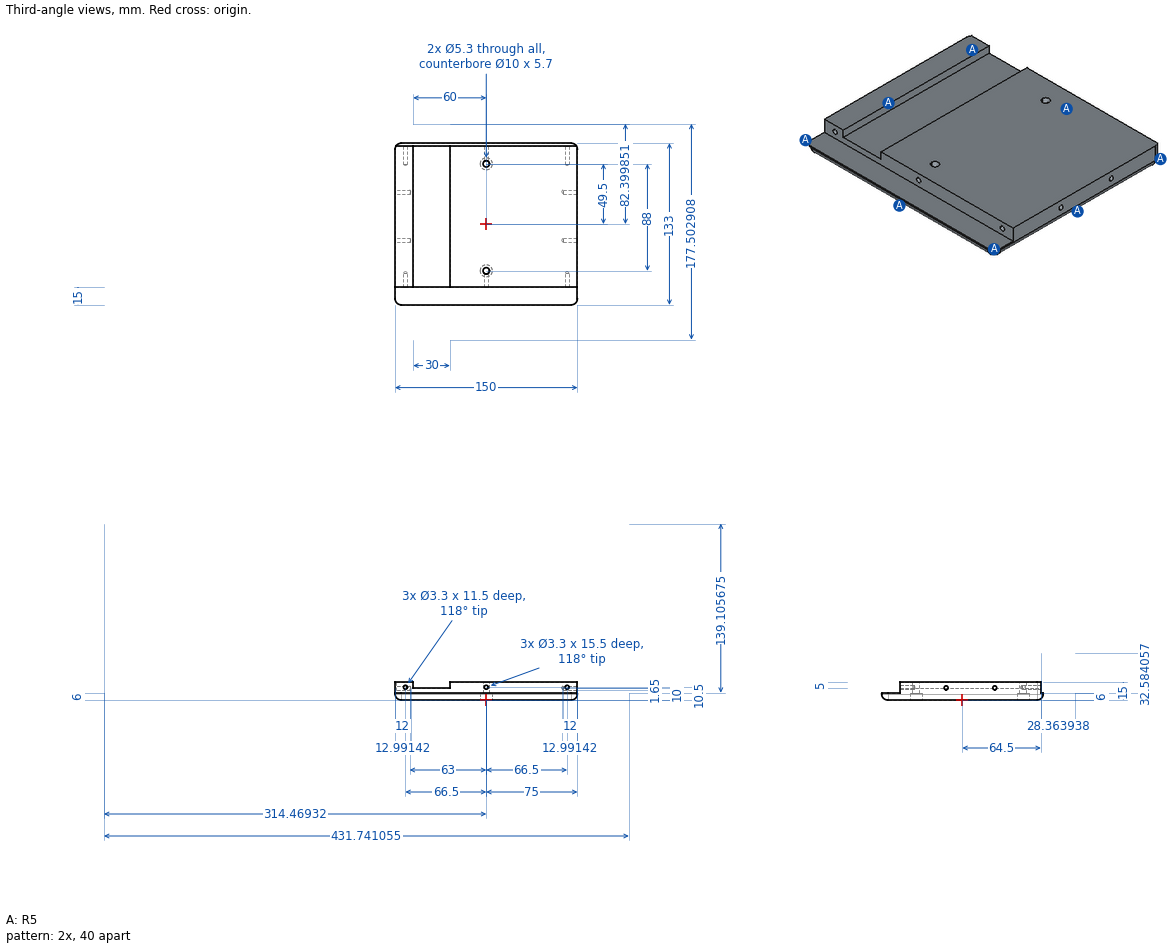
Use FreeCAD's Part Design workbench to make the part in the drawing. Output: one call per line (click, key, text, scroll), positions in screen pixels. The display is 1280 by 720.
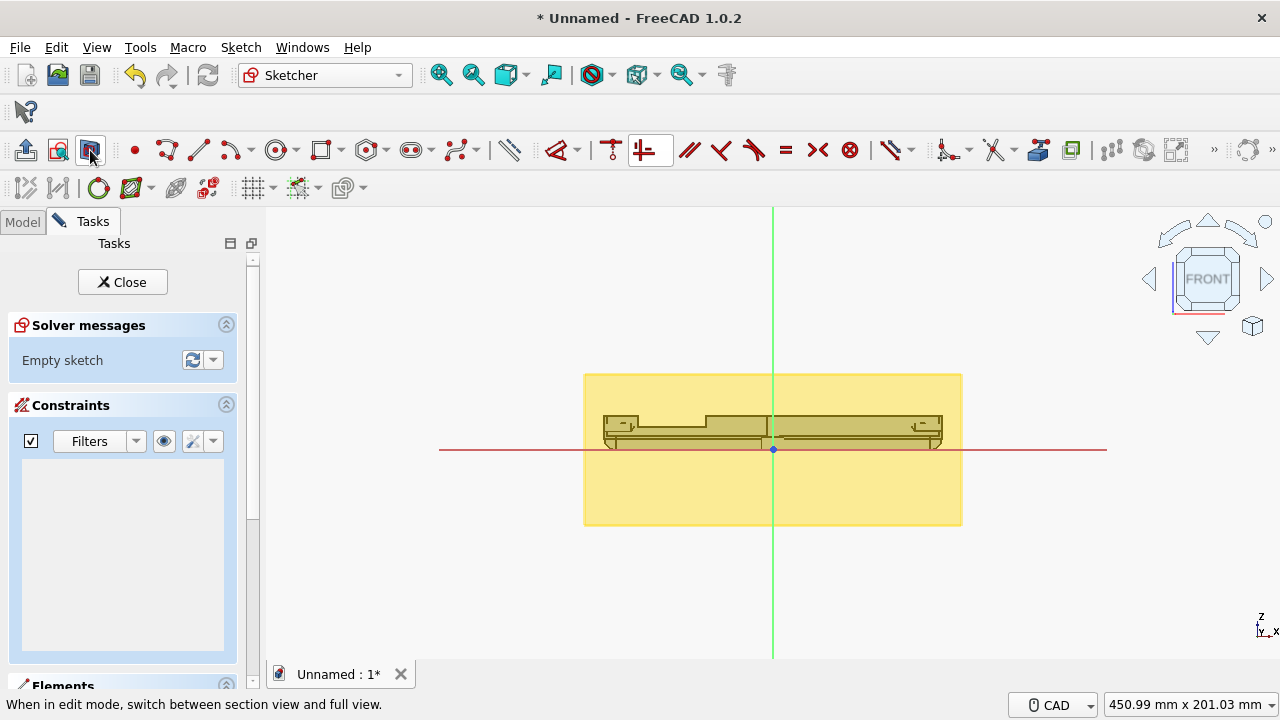
scroll(606, 429, up, 13)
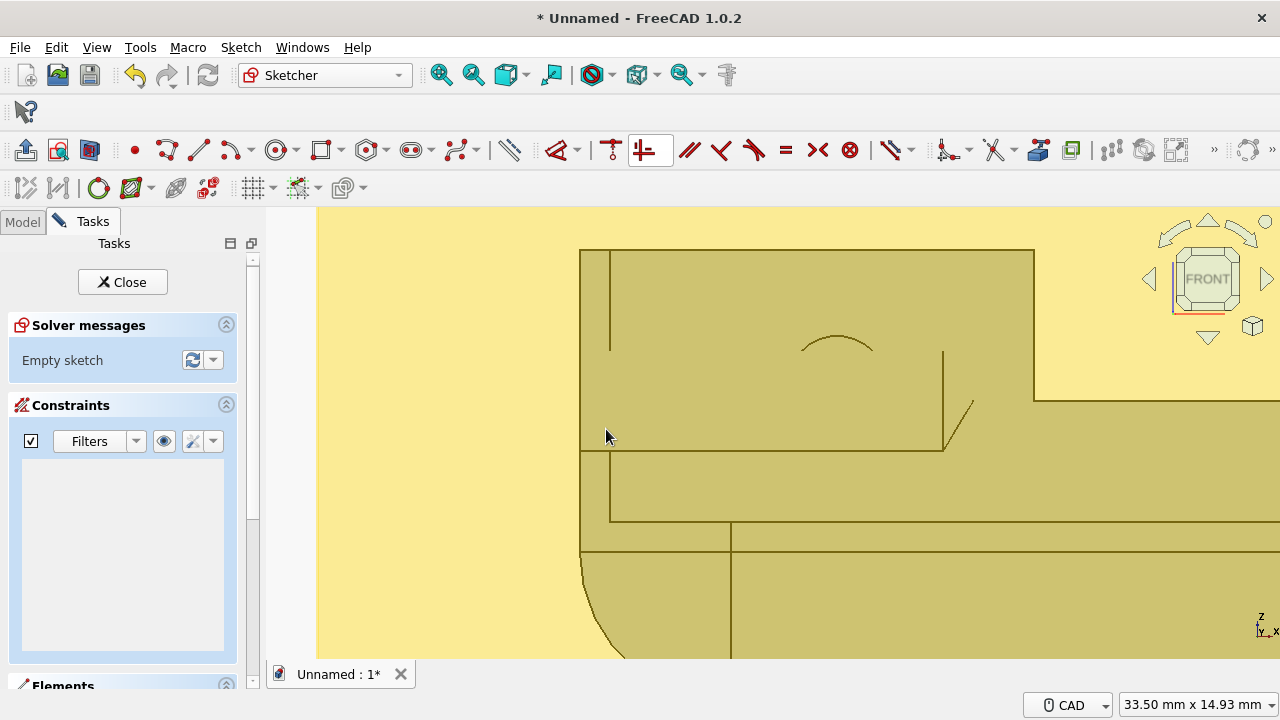
click(168, 150)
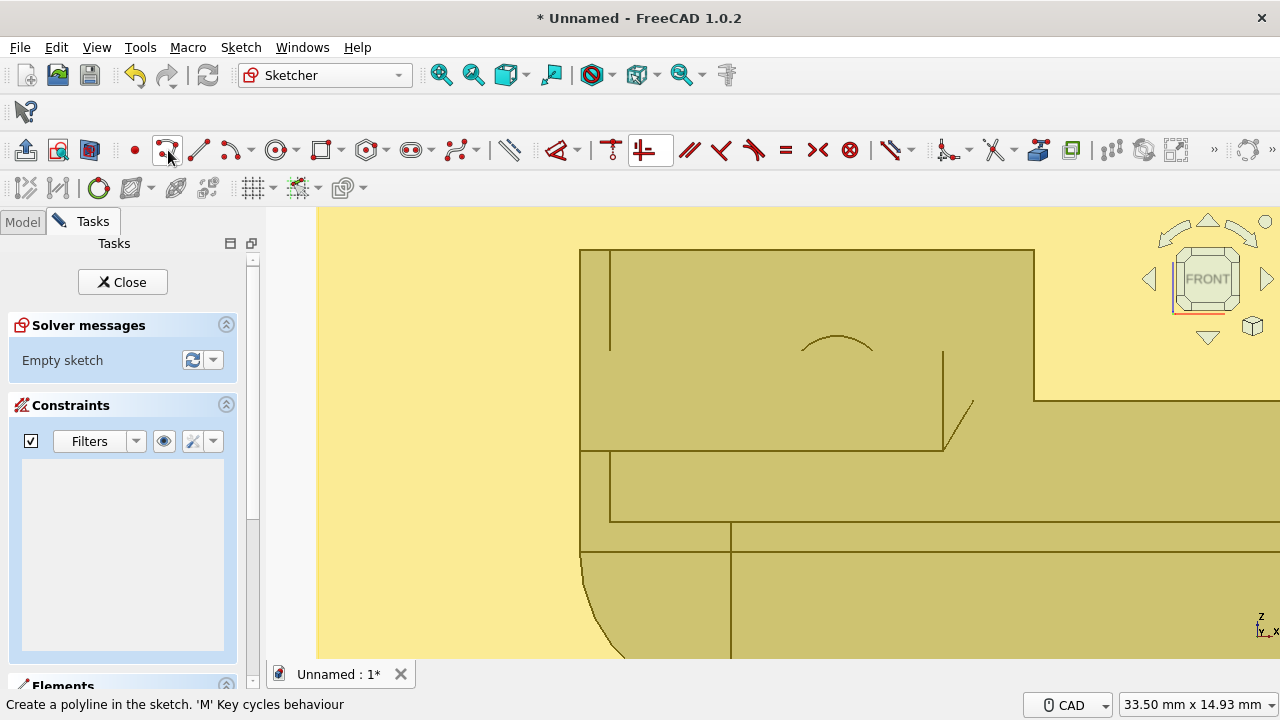
click(973, 401)
click(943, 451)
click(580, 451)
click(580, 401)
click(973, 402)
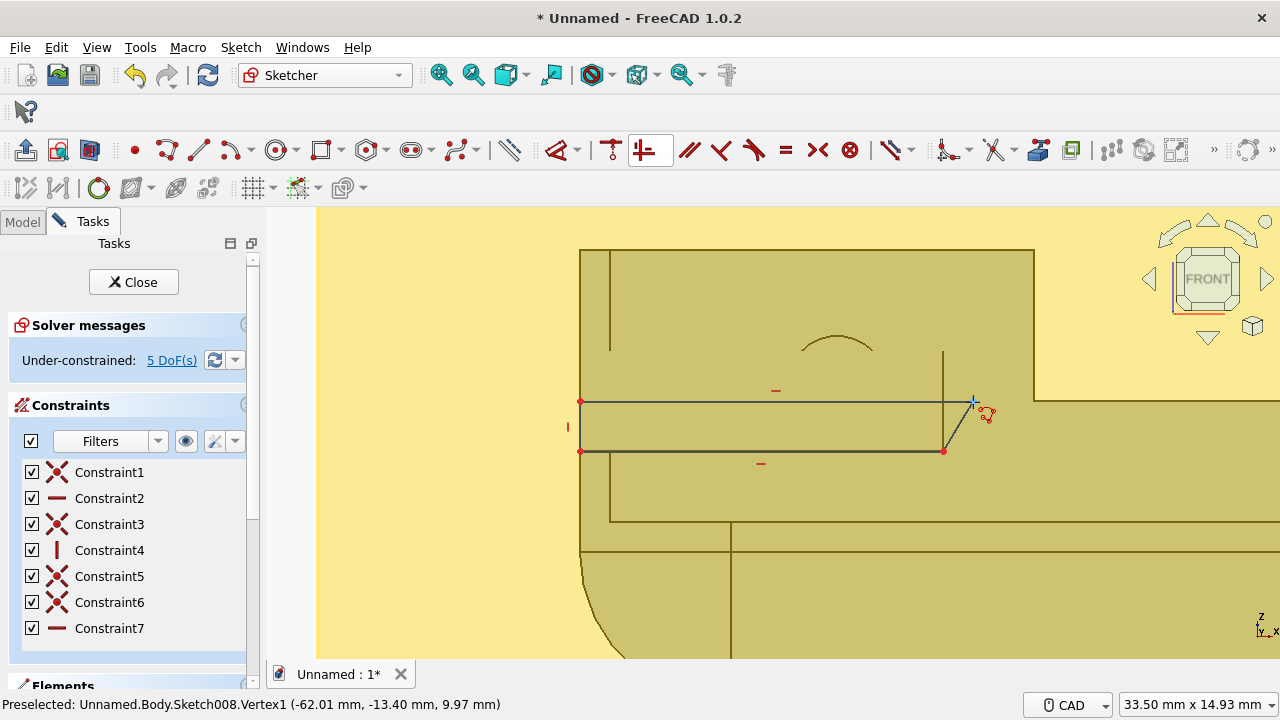
click(200, 150)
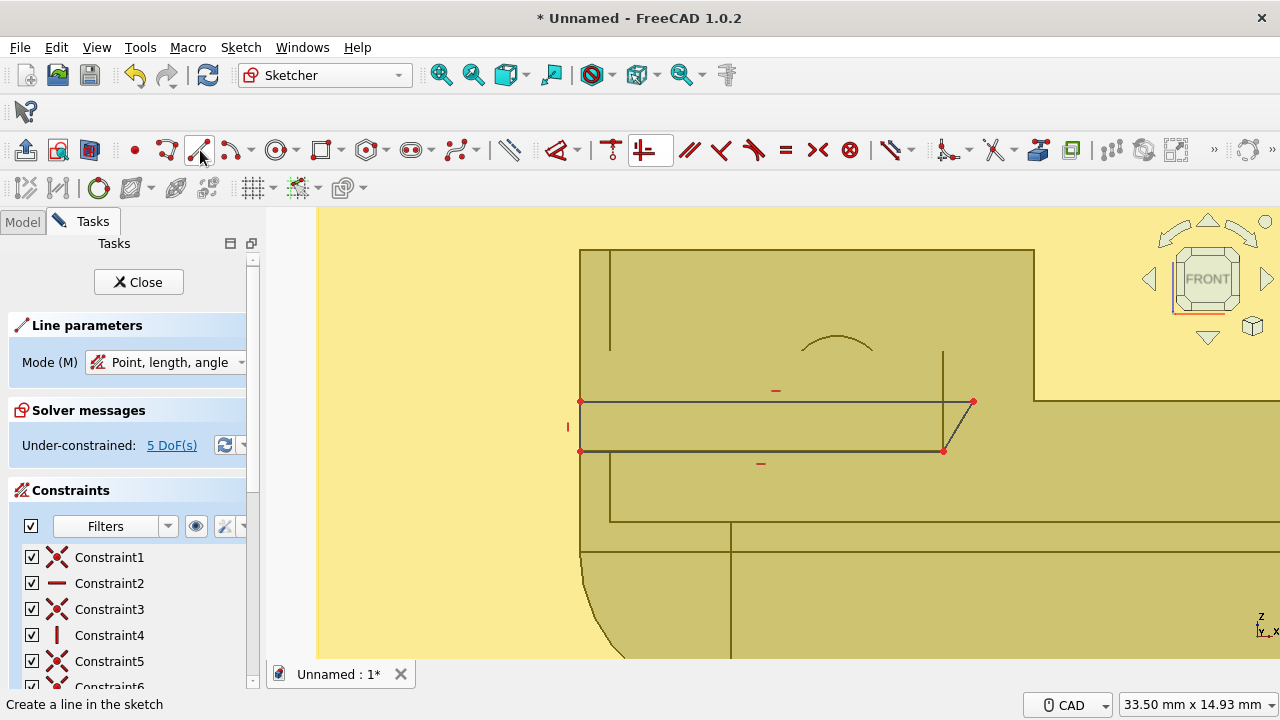
click(541, 401)
click(423, 401)
key(Escape)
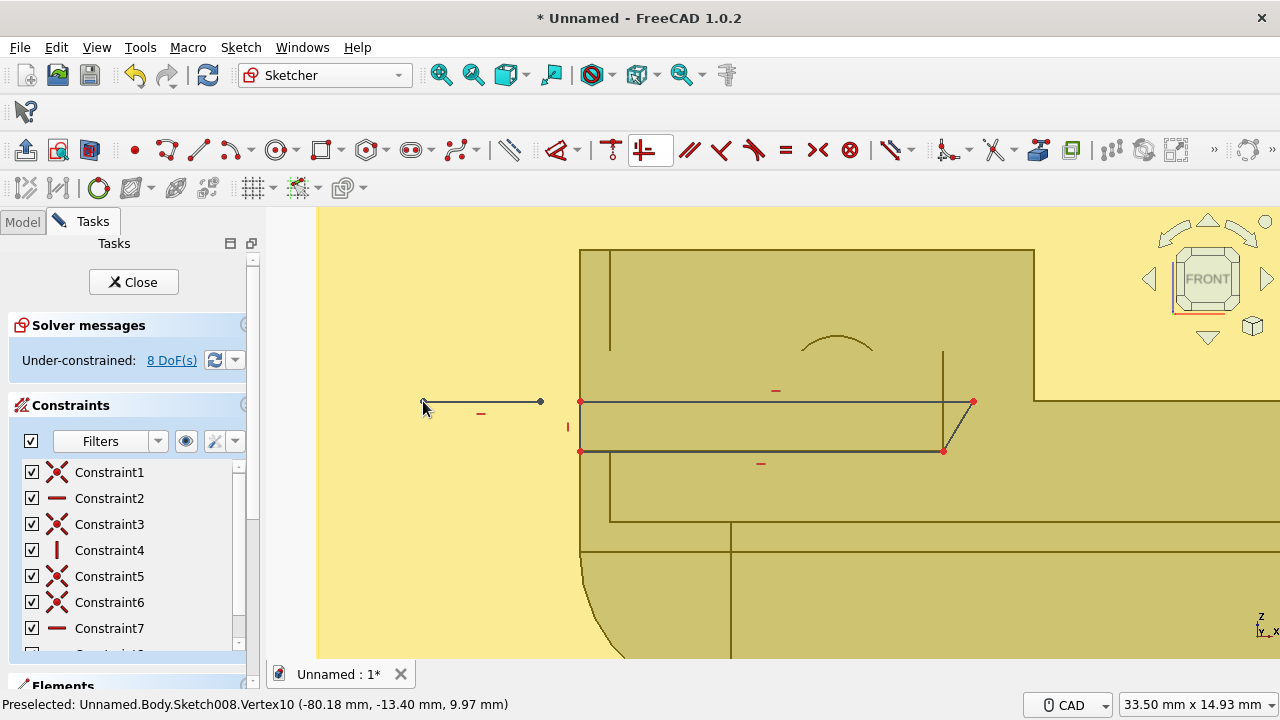
click(506, 402)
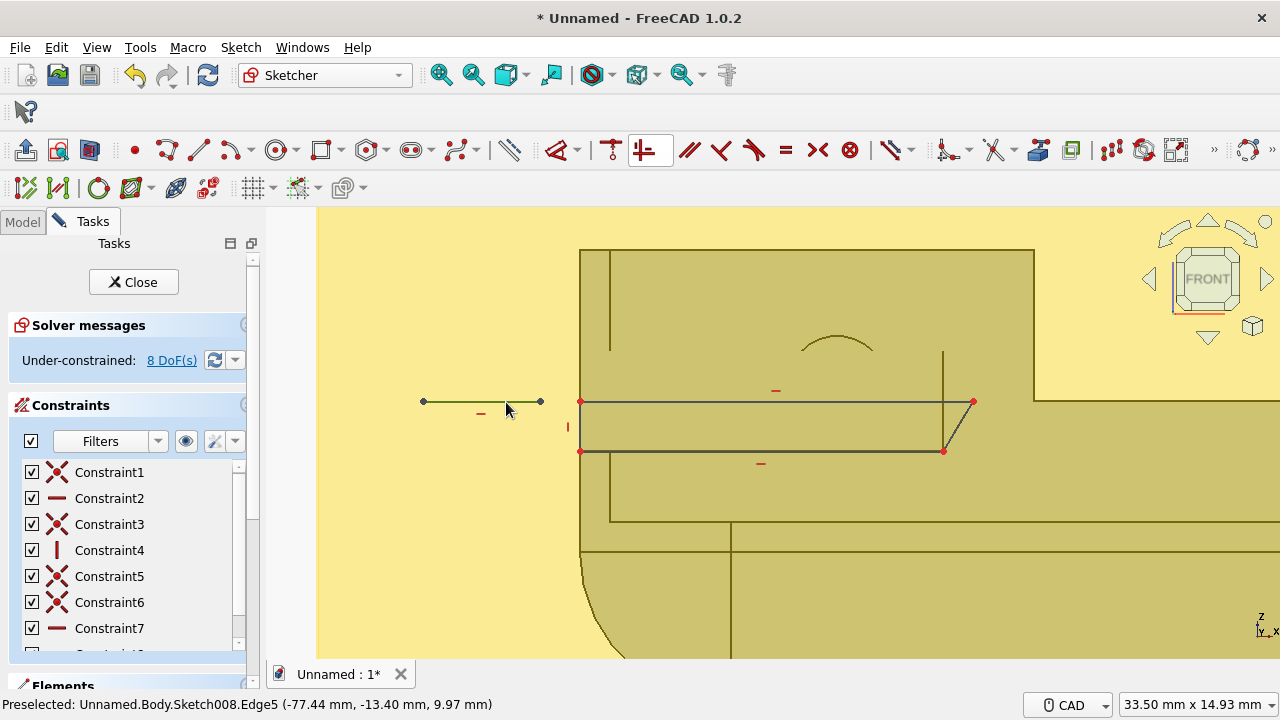
click(510, 150)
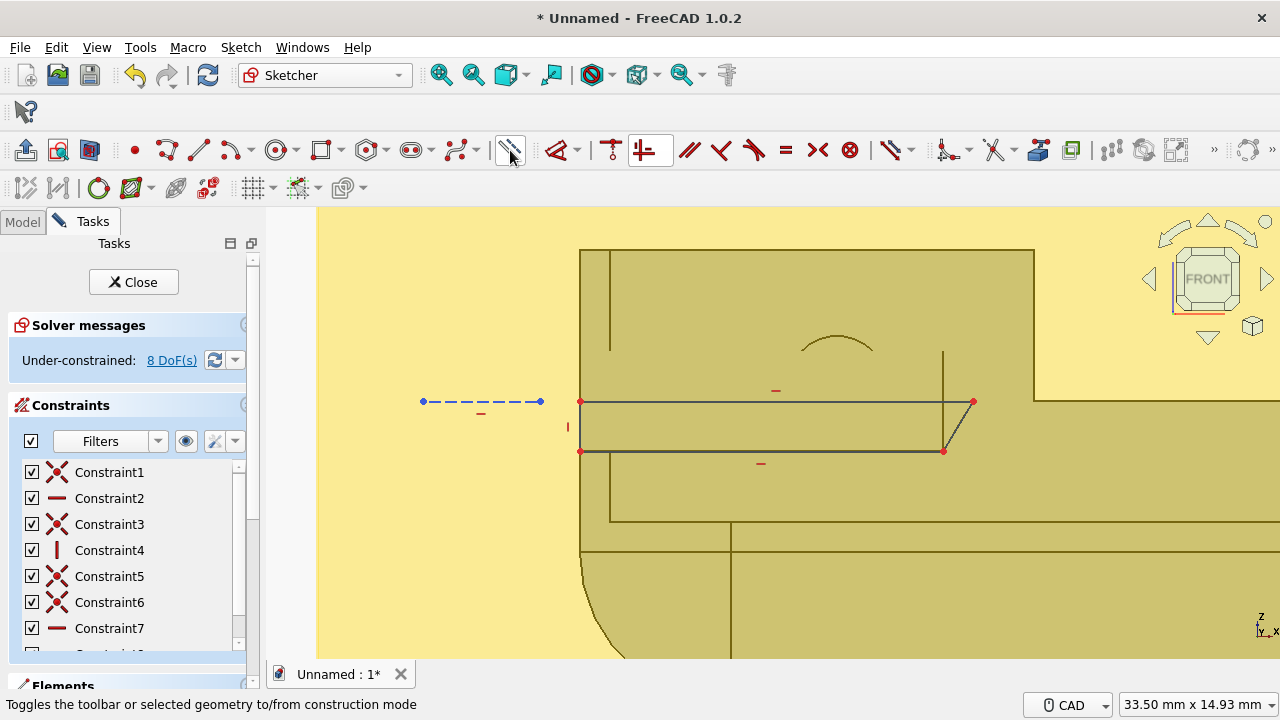
click(556, 150)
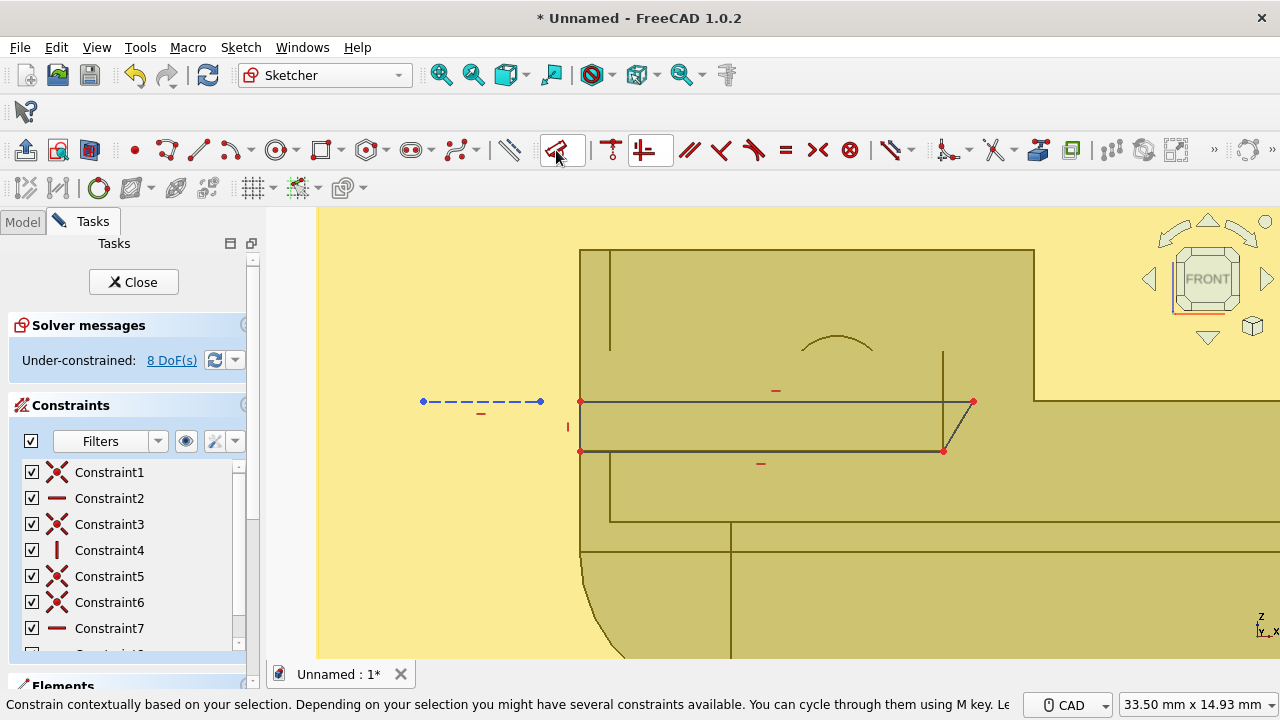
click(834, 452)
click(761, 486)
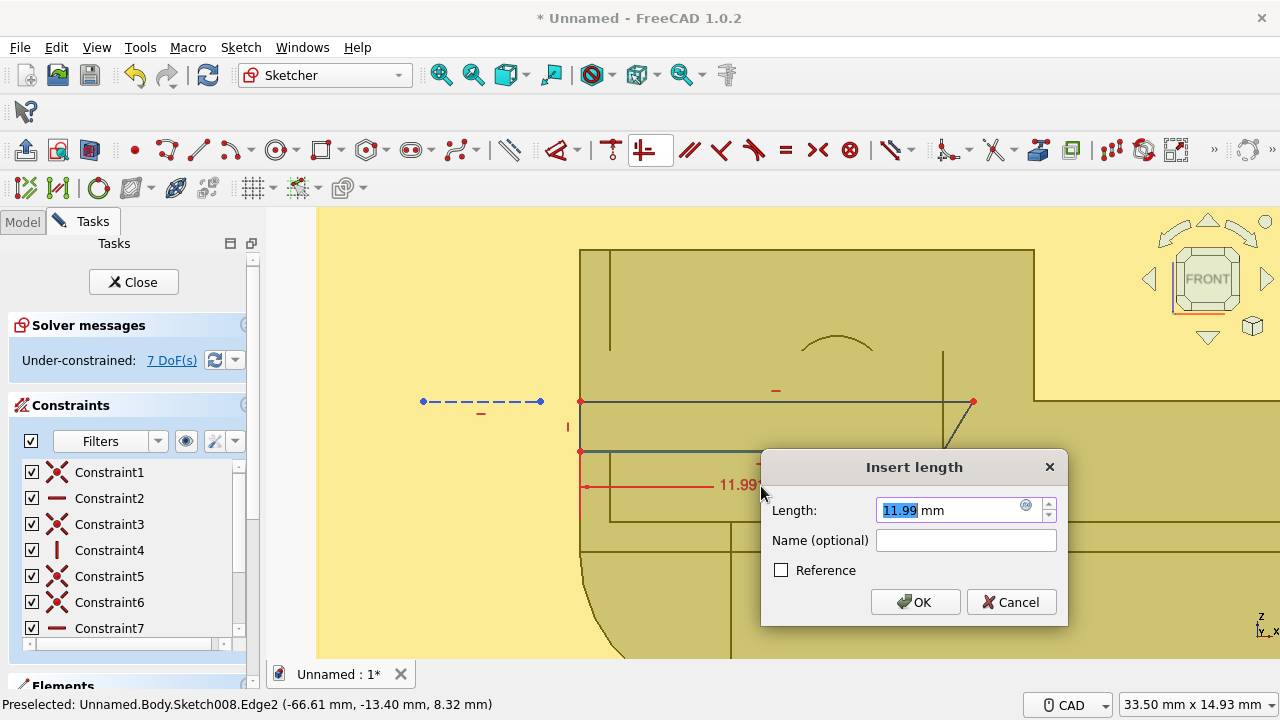
text(12)
key(Return)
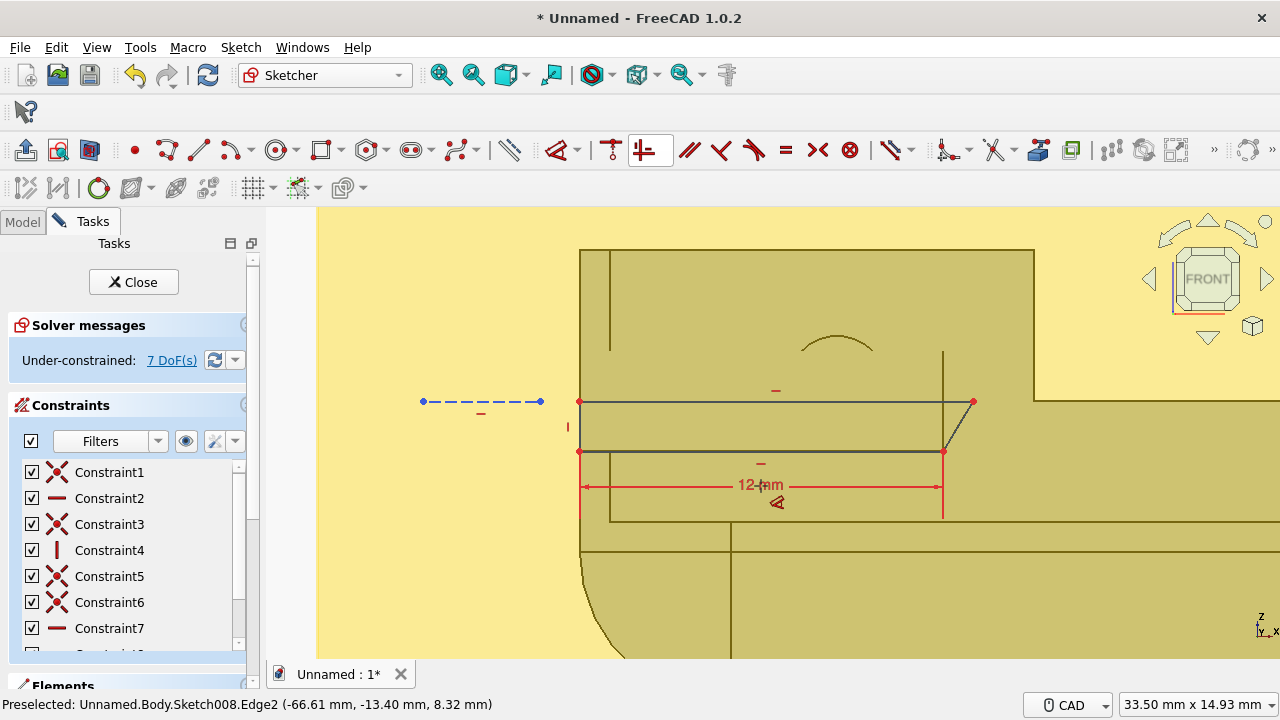
click(973, 402)
click(939, 516)